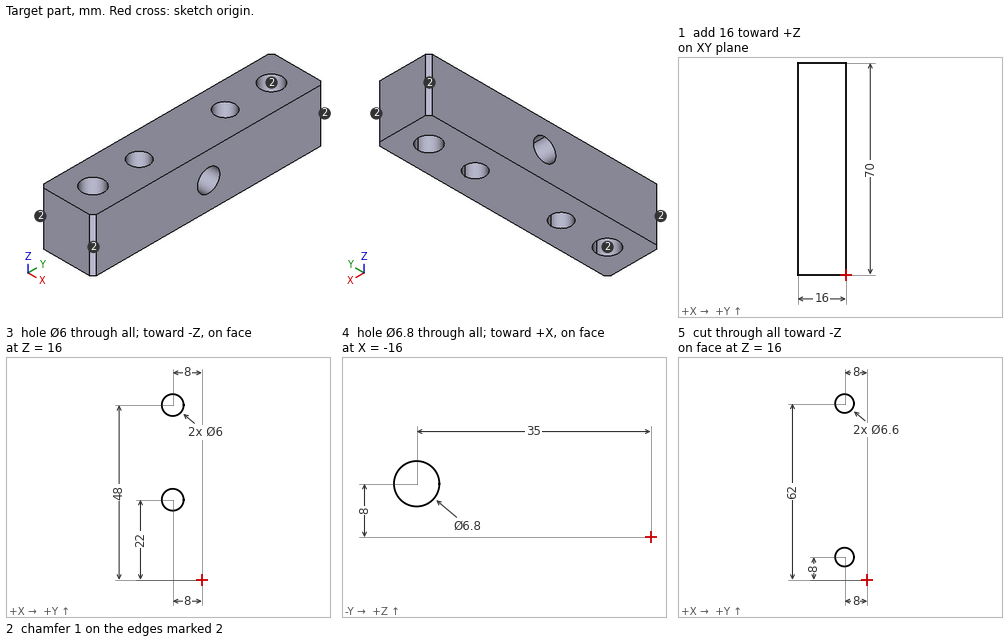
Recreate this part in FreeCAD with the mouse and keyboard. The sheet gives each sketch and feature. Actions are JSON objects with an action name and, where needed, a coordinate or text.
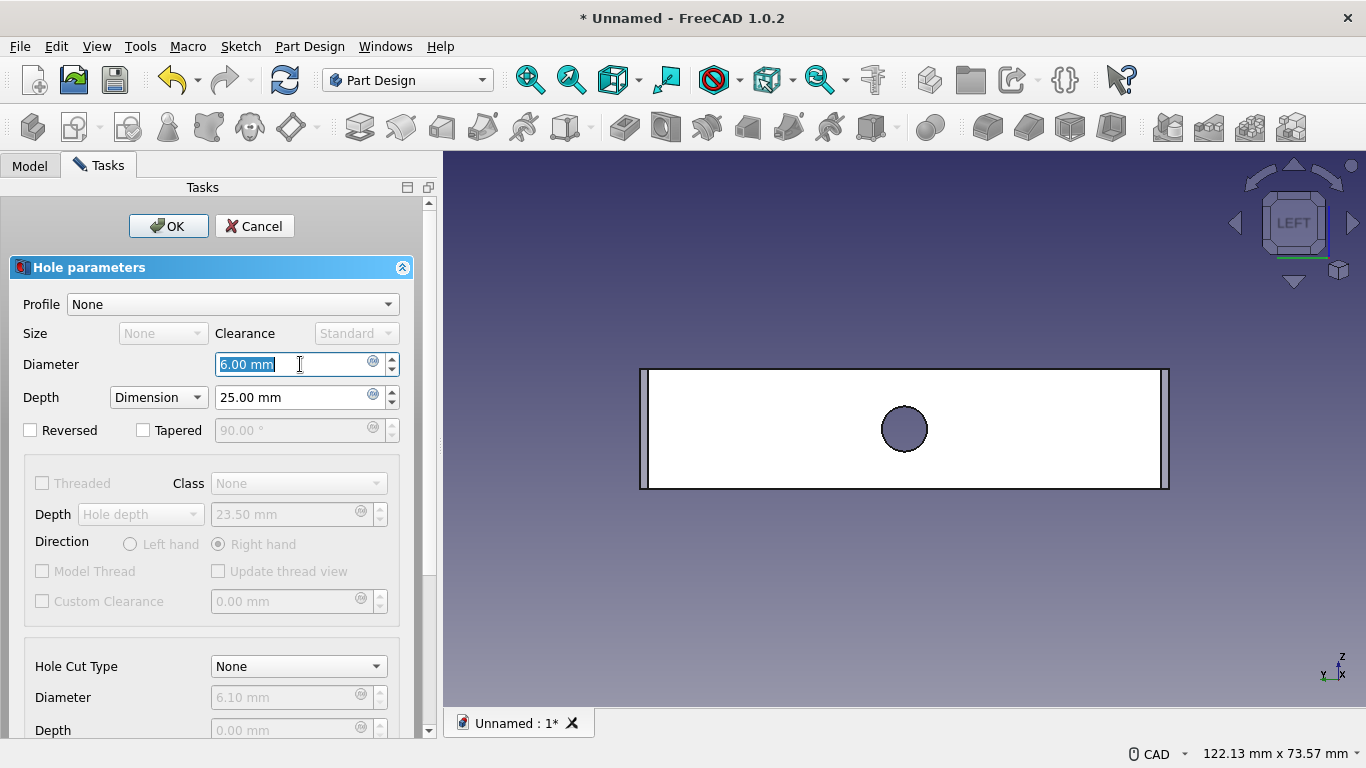
{"action": "type", "text": "6.8"}
{"action": "key", "text": "Tab"}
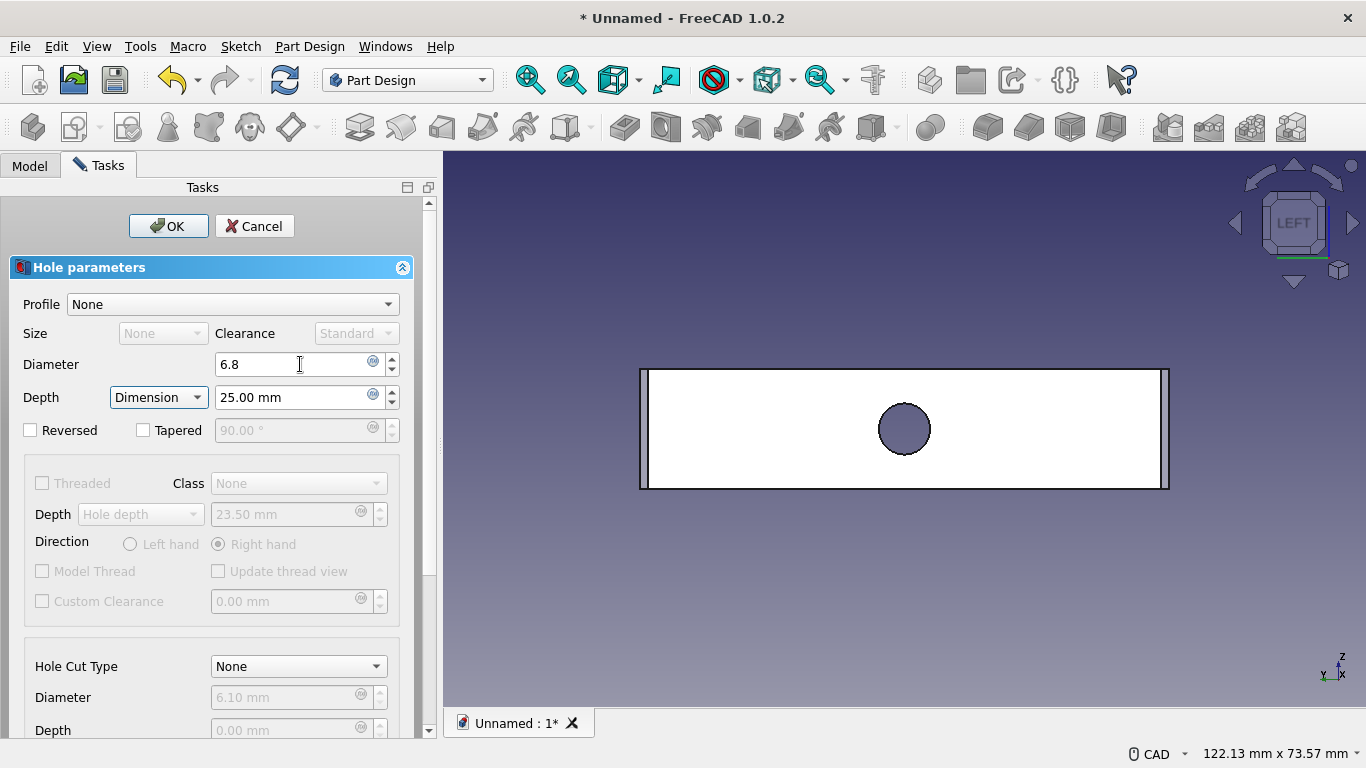
{"action": "left_click", "coordinate": [160, 398]}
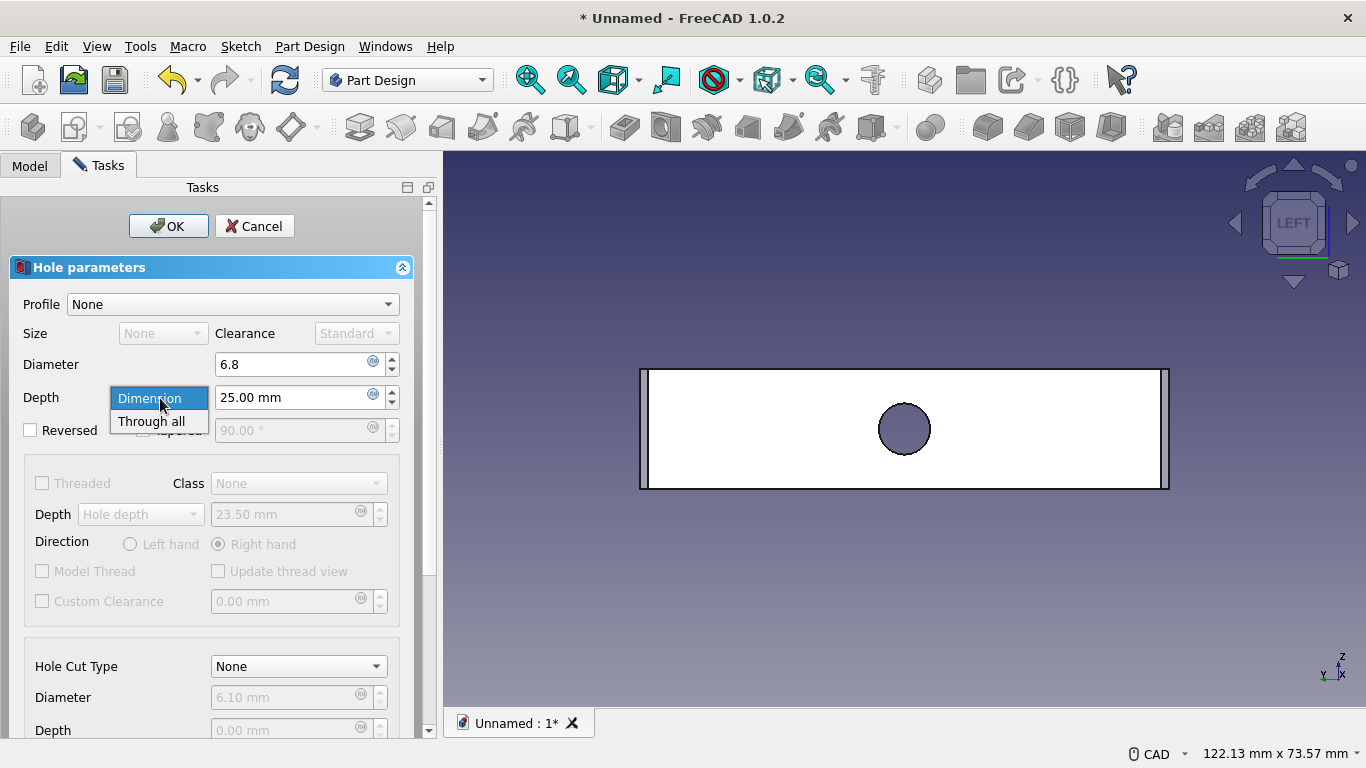
{"action": "left_click", "coordinate": [158, 422]}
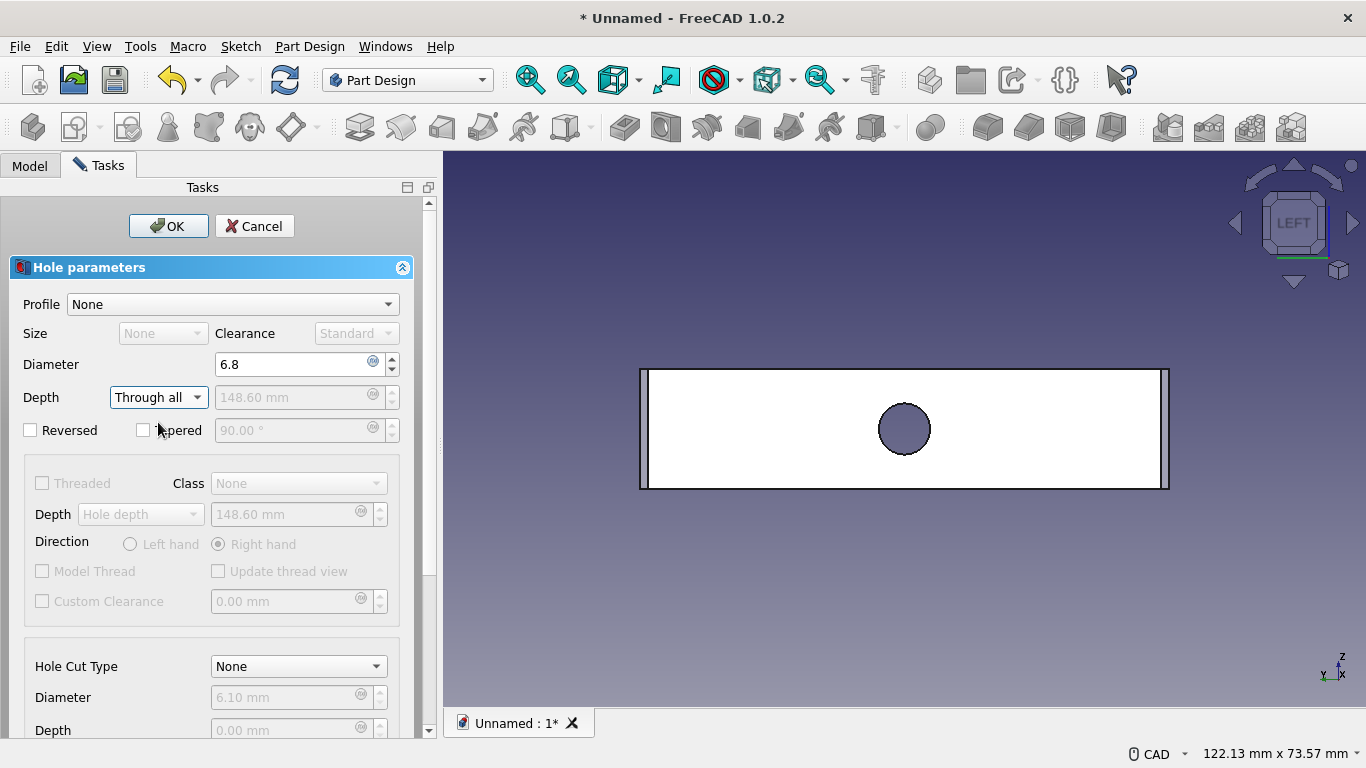
{"action": "left_click", "coordinate": [169, 226]}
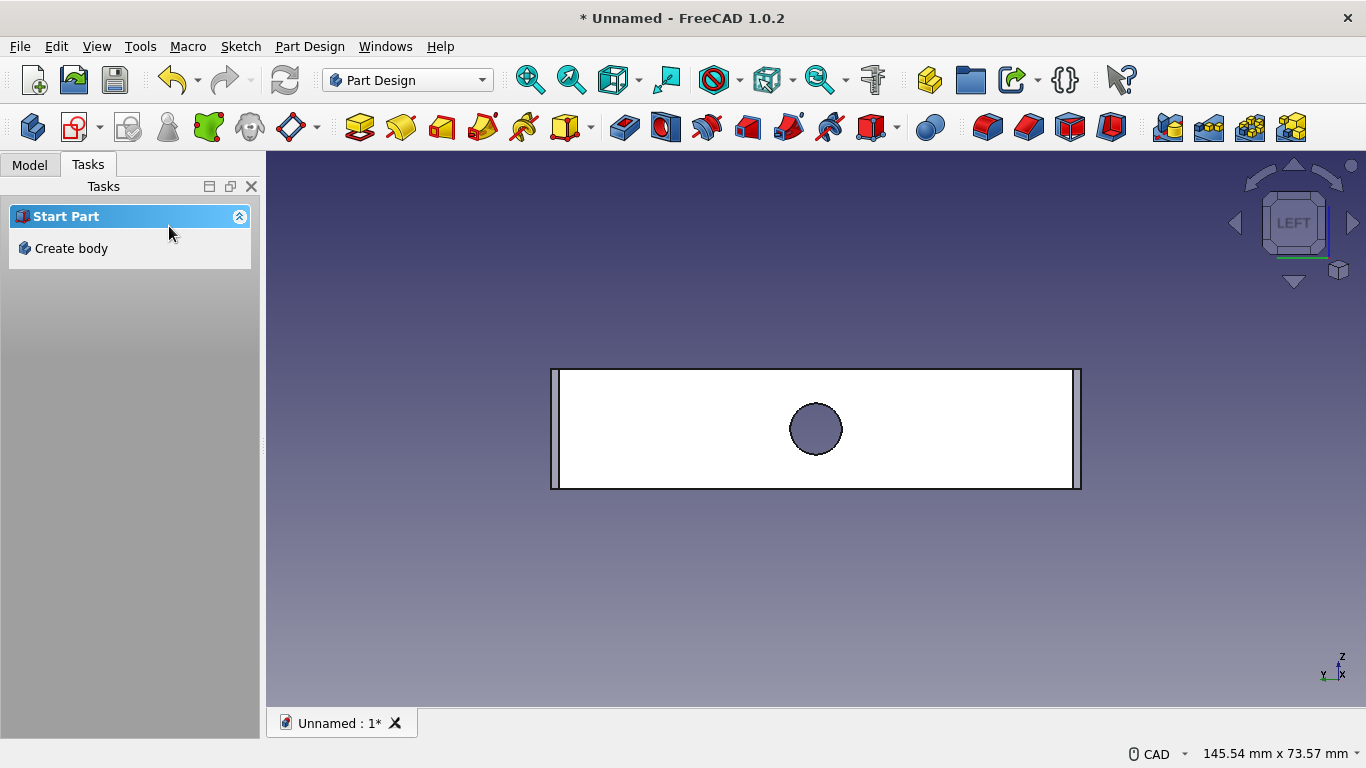
{"action": "key", "text": "0"}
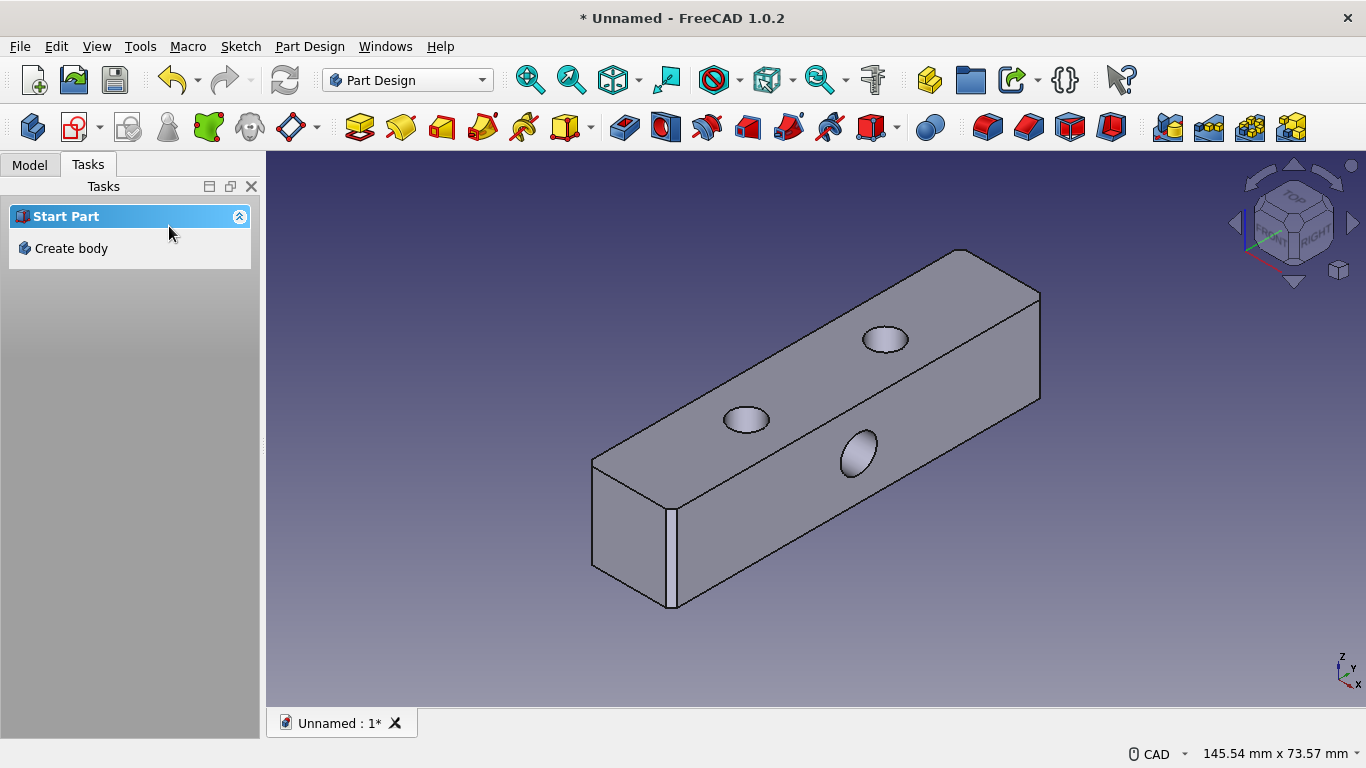
{"action": "left_click", "coordinate": [816, 379]}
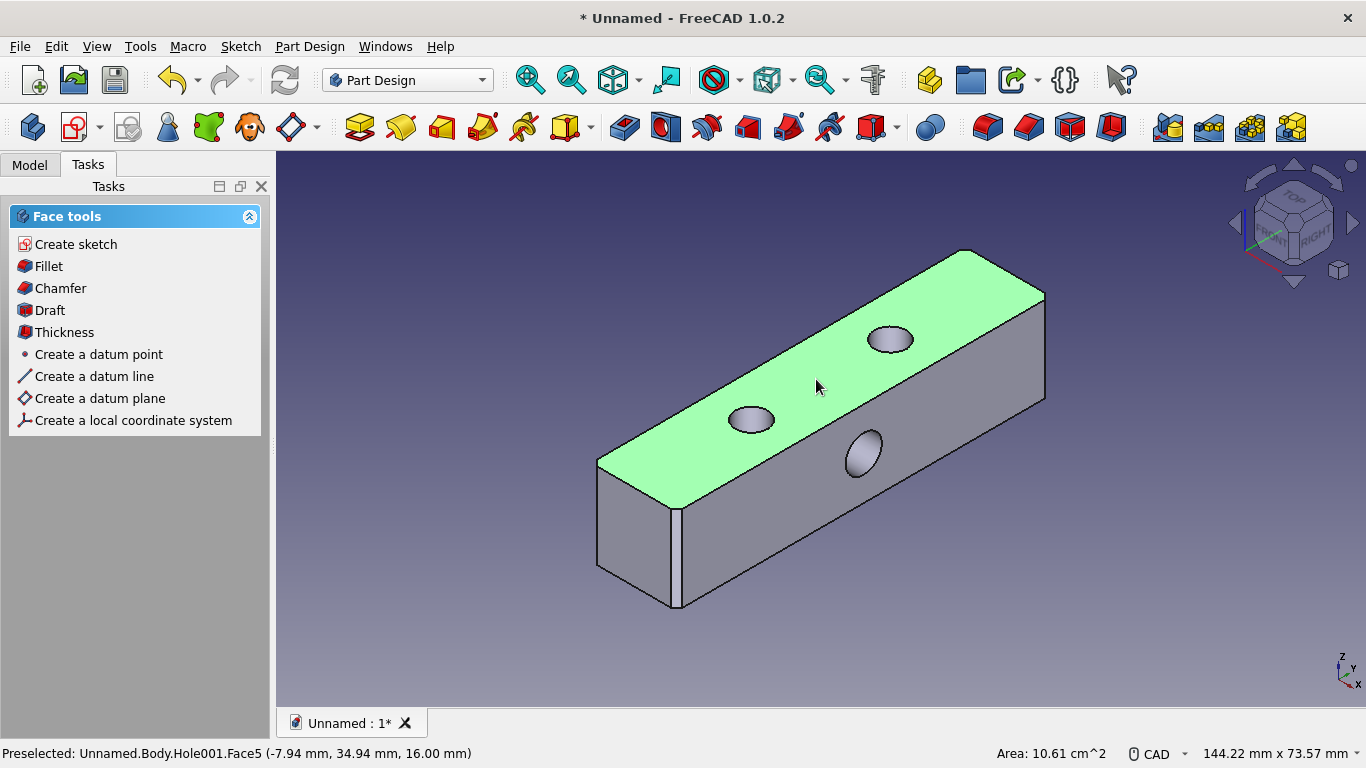
{"action": "left_click", "coordinate": [74, 128]}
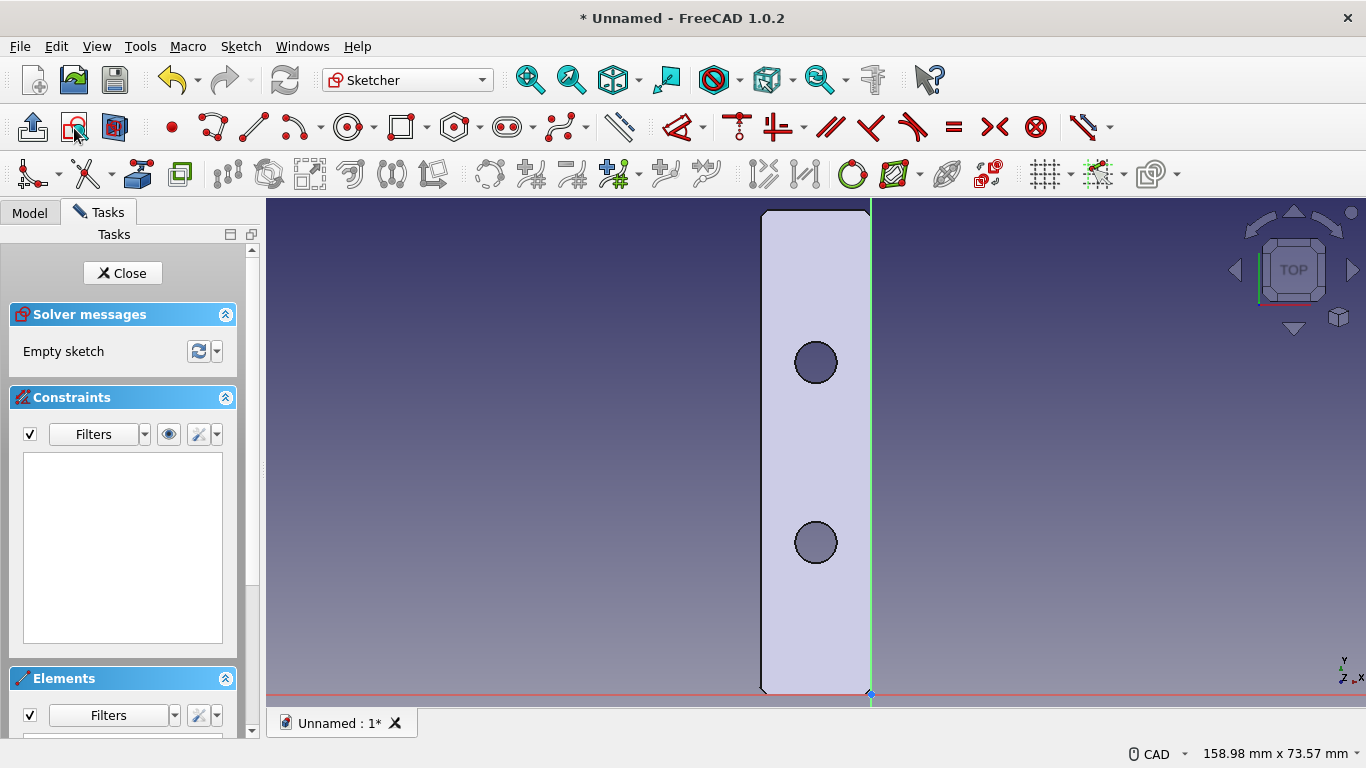
{"action": "scroll", "coordinate": [575, 419], "scroll_direction": "down", "scroll_amount": 2}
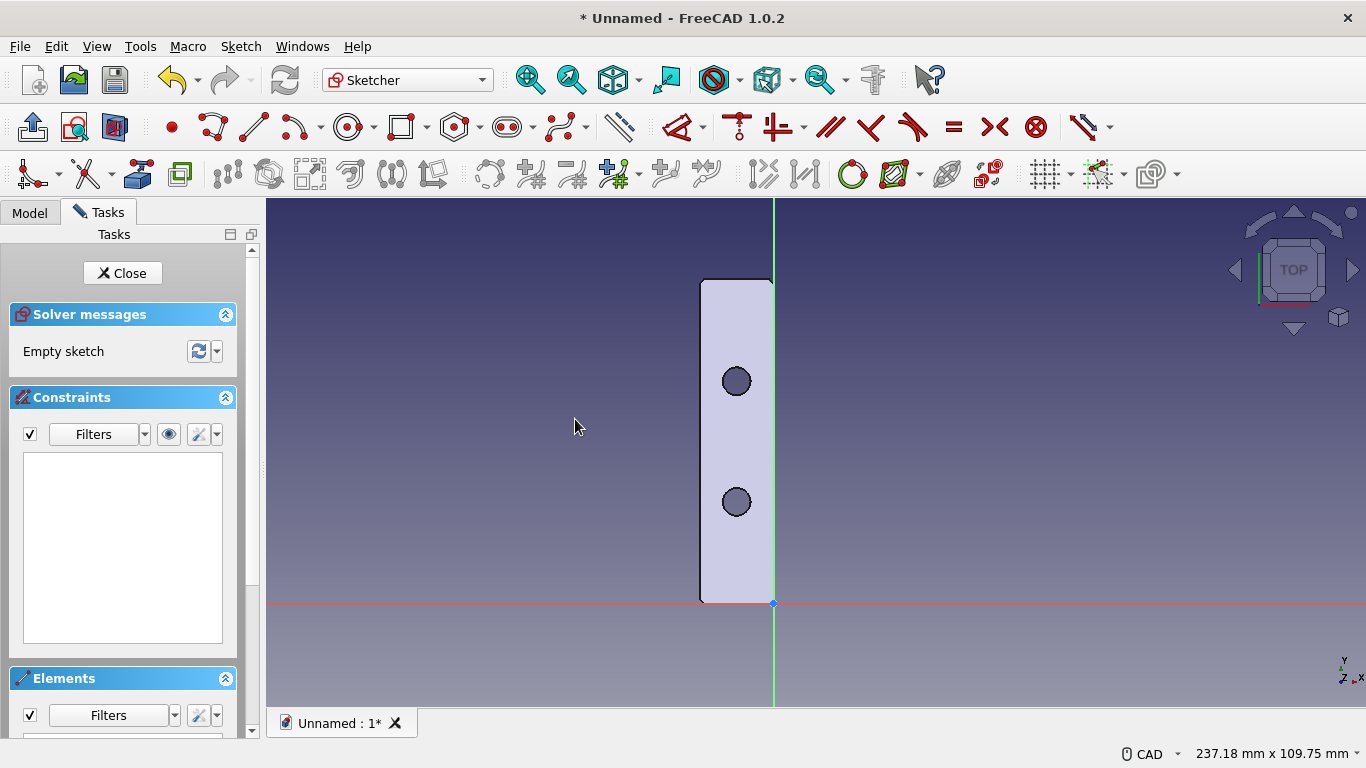
{"action": "left_click", "coordinate": [348, 128]}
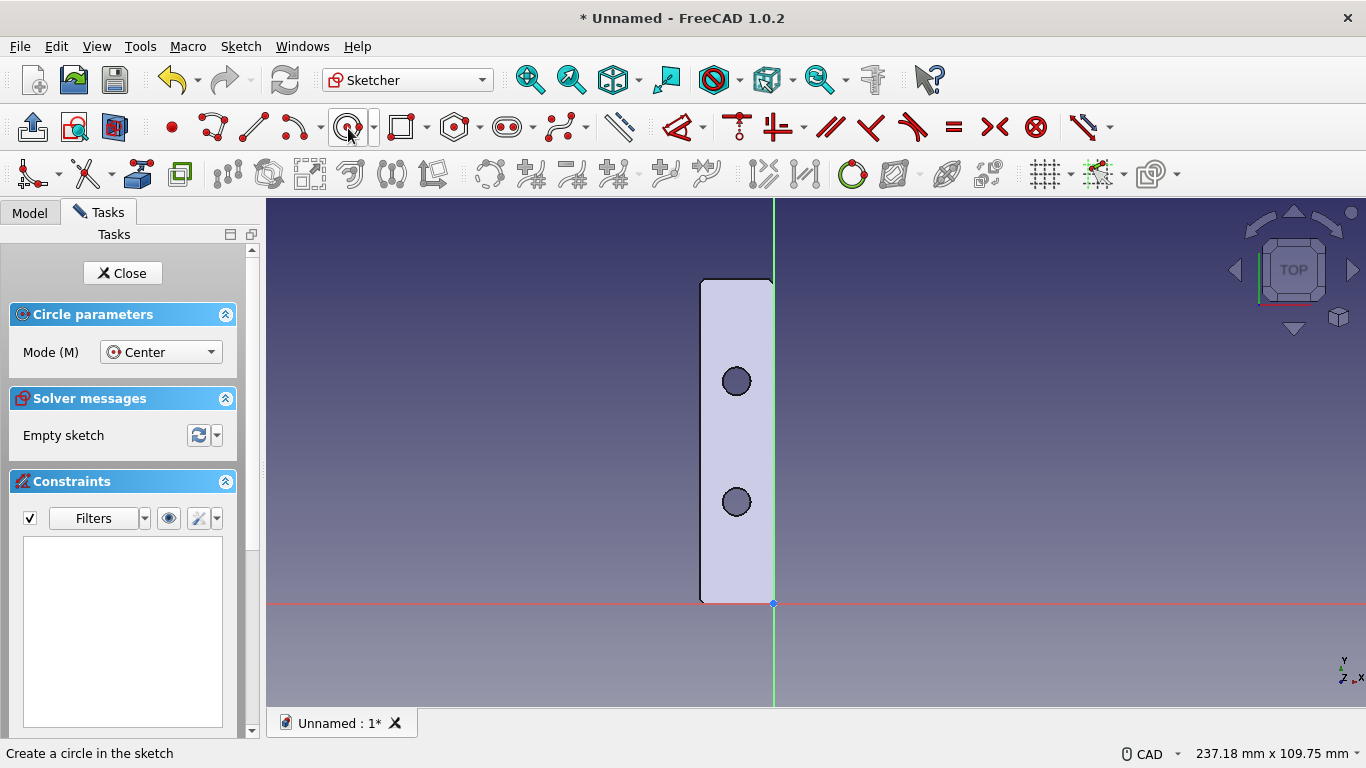
{"action": "scroll", "coordinate": [737, 316], "scroll_direction": "up", "scroll_amount": 2}